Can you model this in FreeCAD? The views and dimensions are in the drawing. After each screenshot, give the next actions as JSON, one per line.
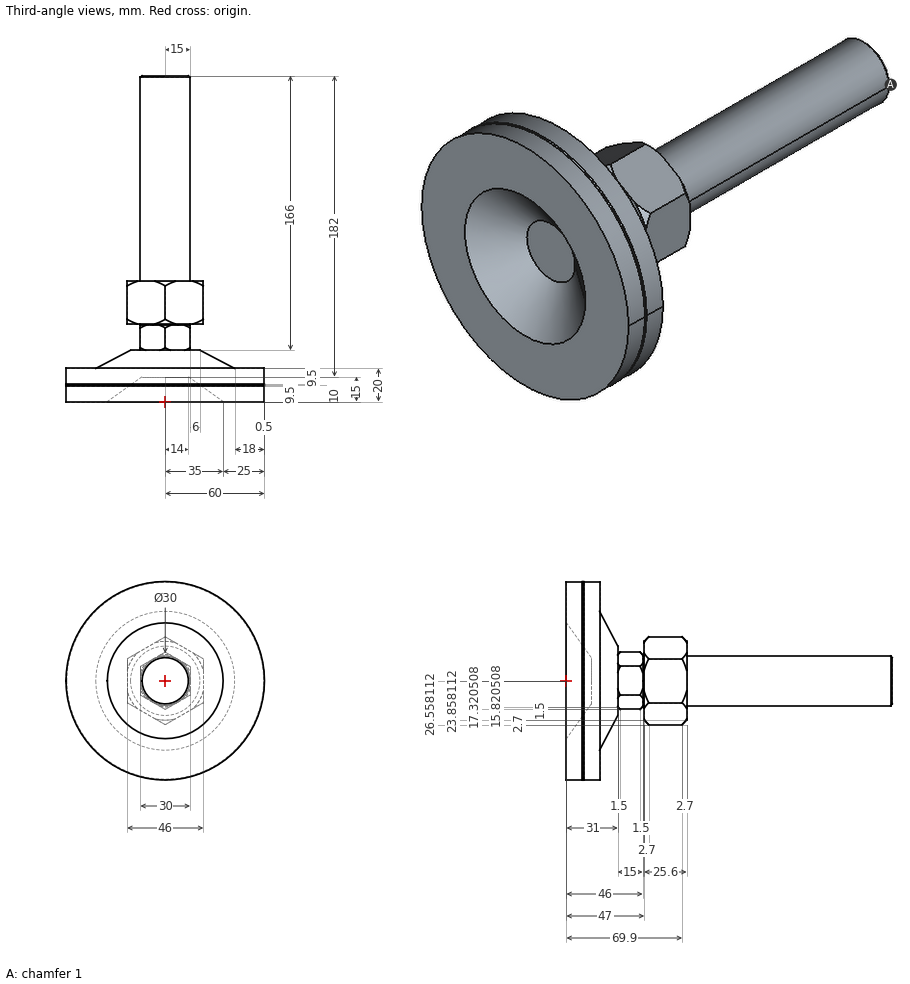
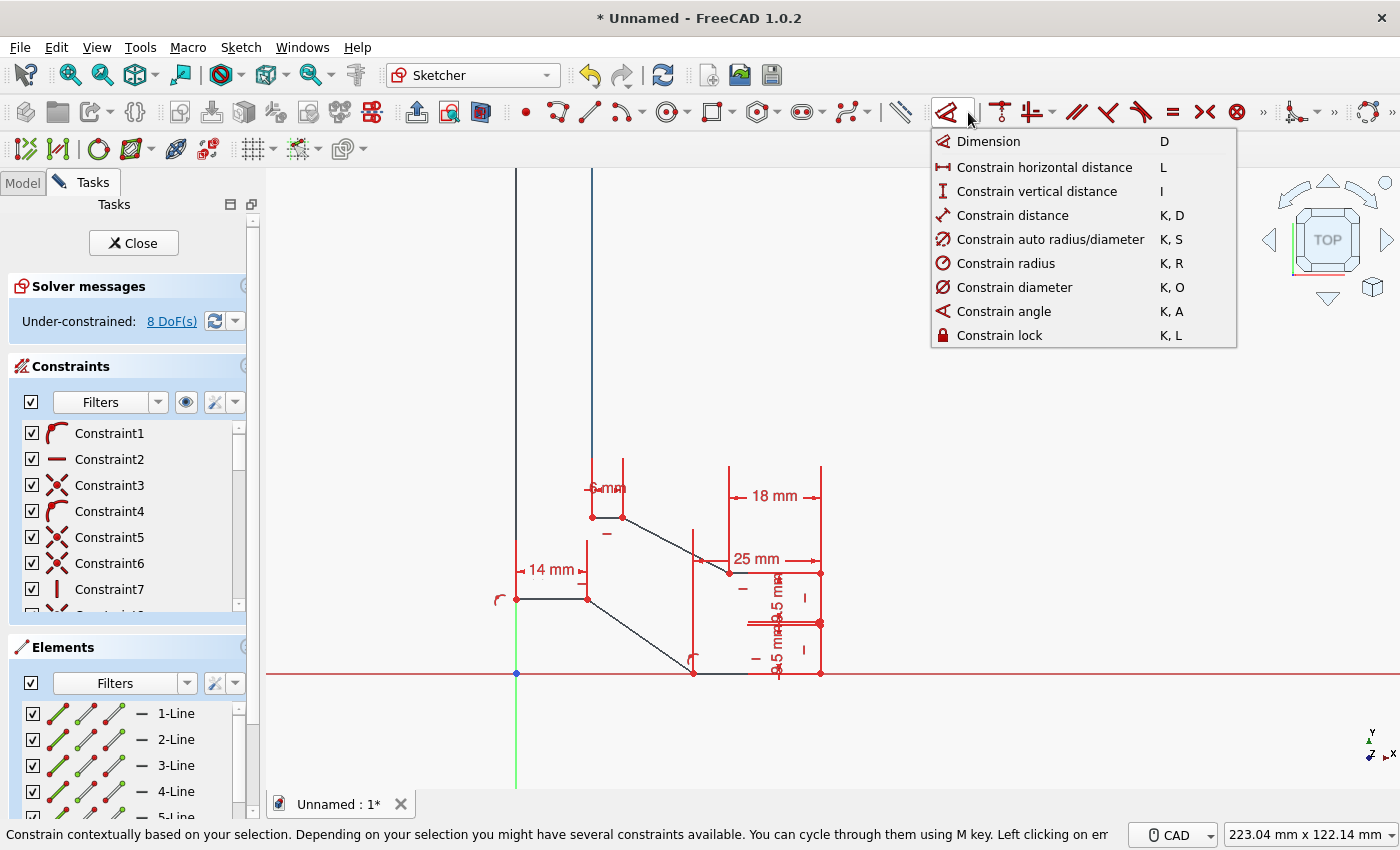
{"action": "left_click", "coordinate": [1084, 191]}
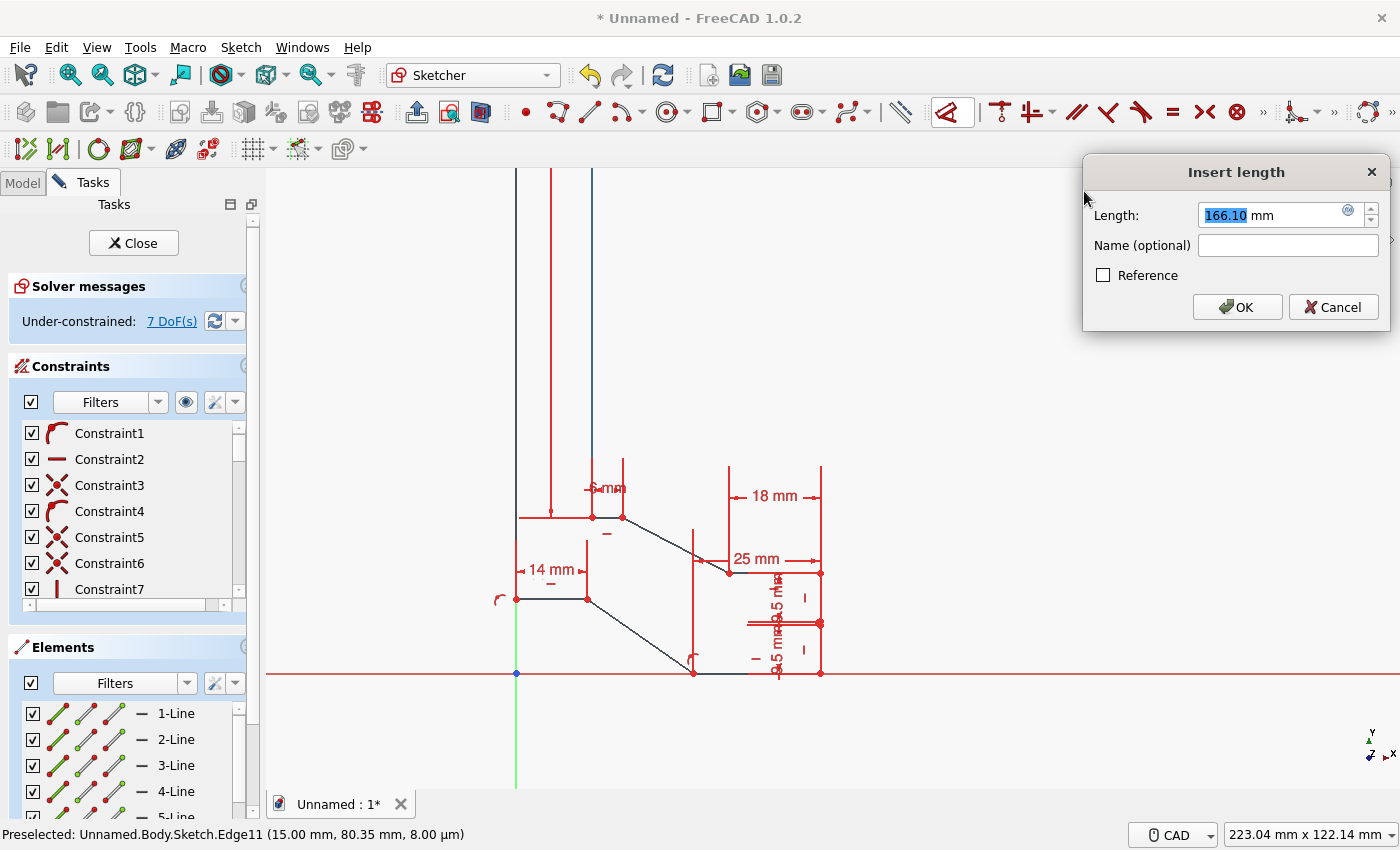
{"action": "type", "text": "166"}
{"action": "key", "text": "Return"}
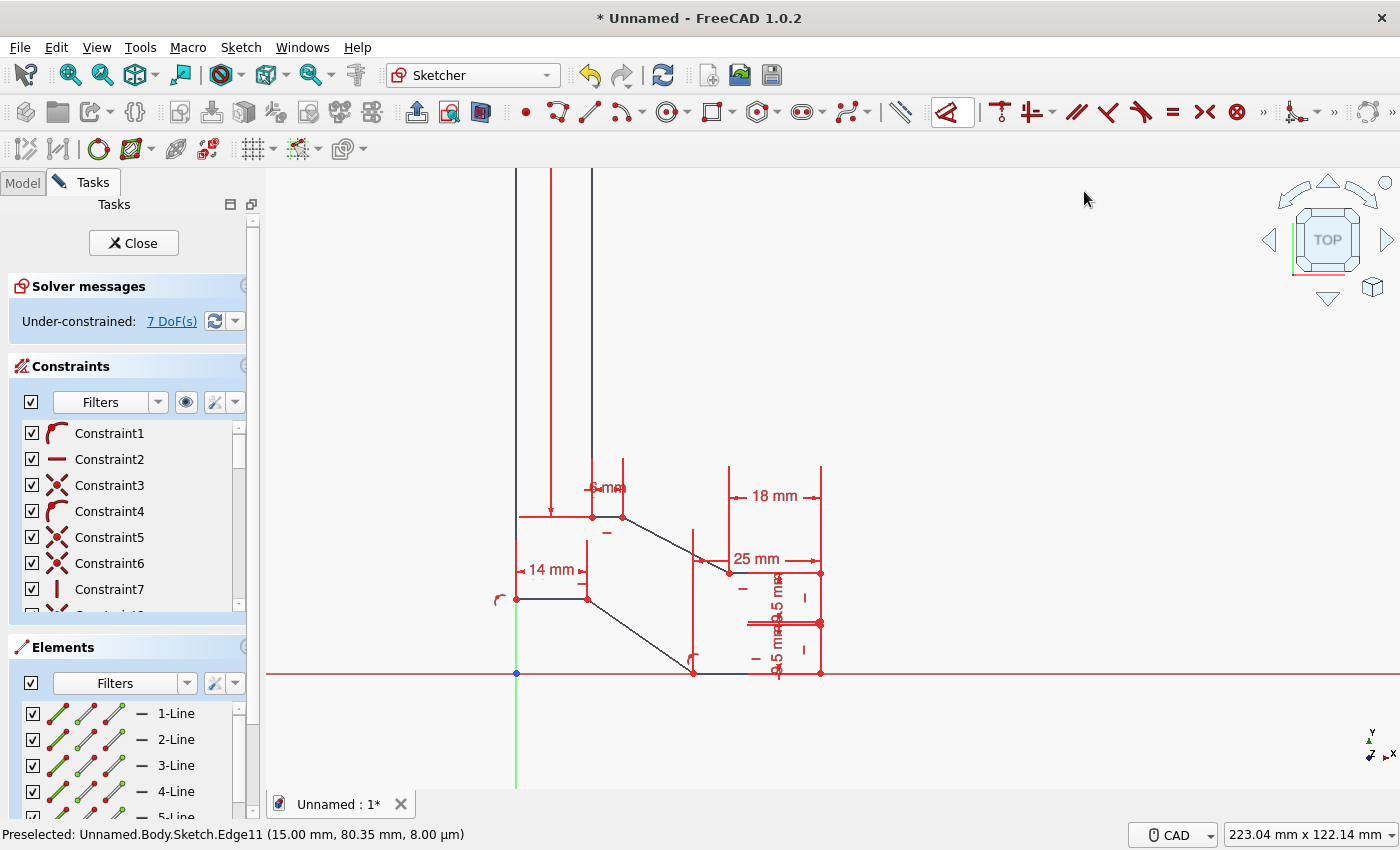
{"action": "left_click", "coordinate": [516, 322]}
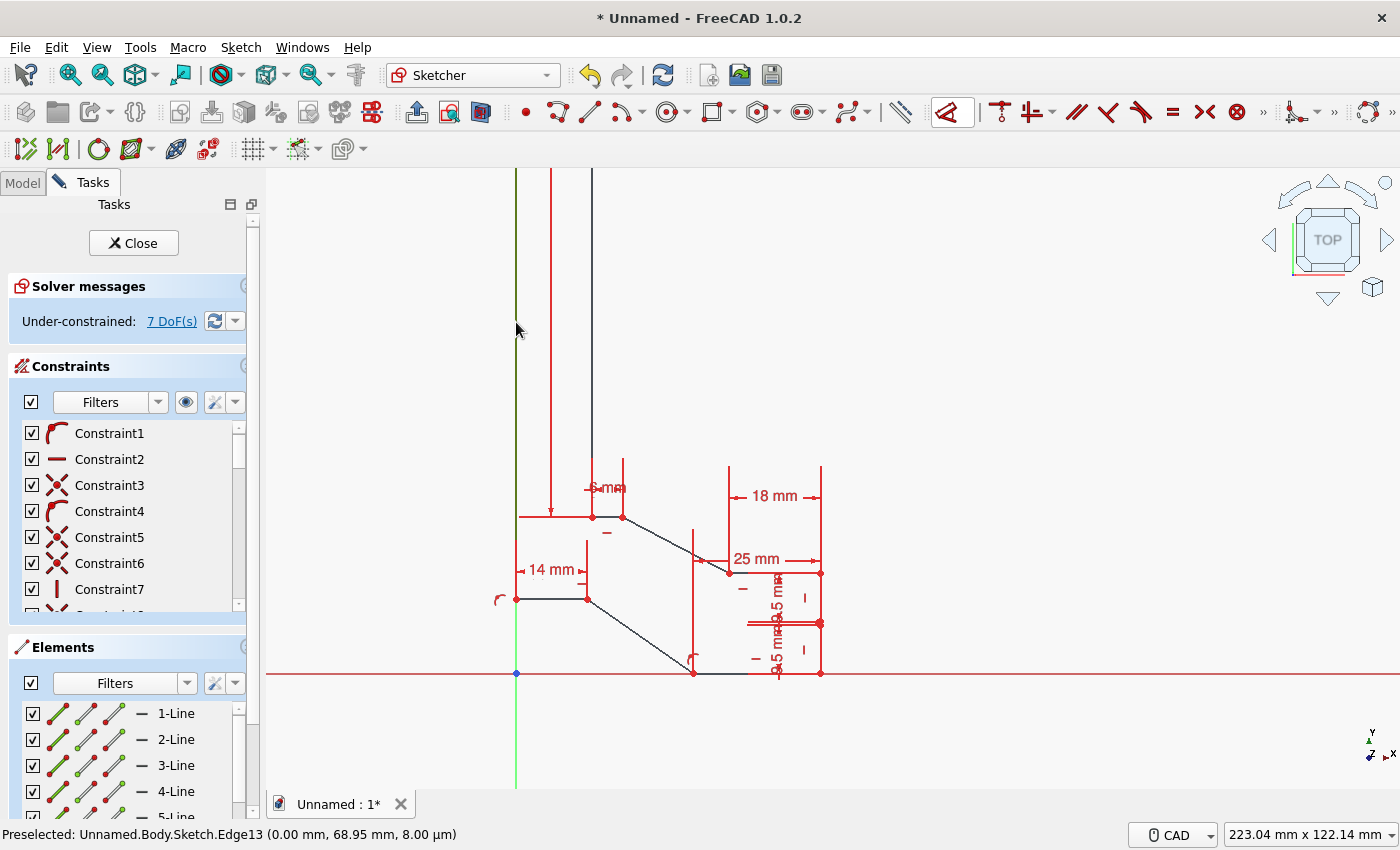
{"action": "key", "text": "i"}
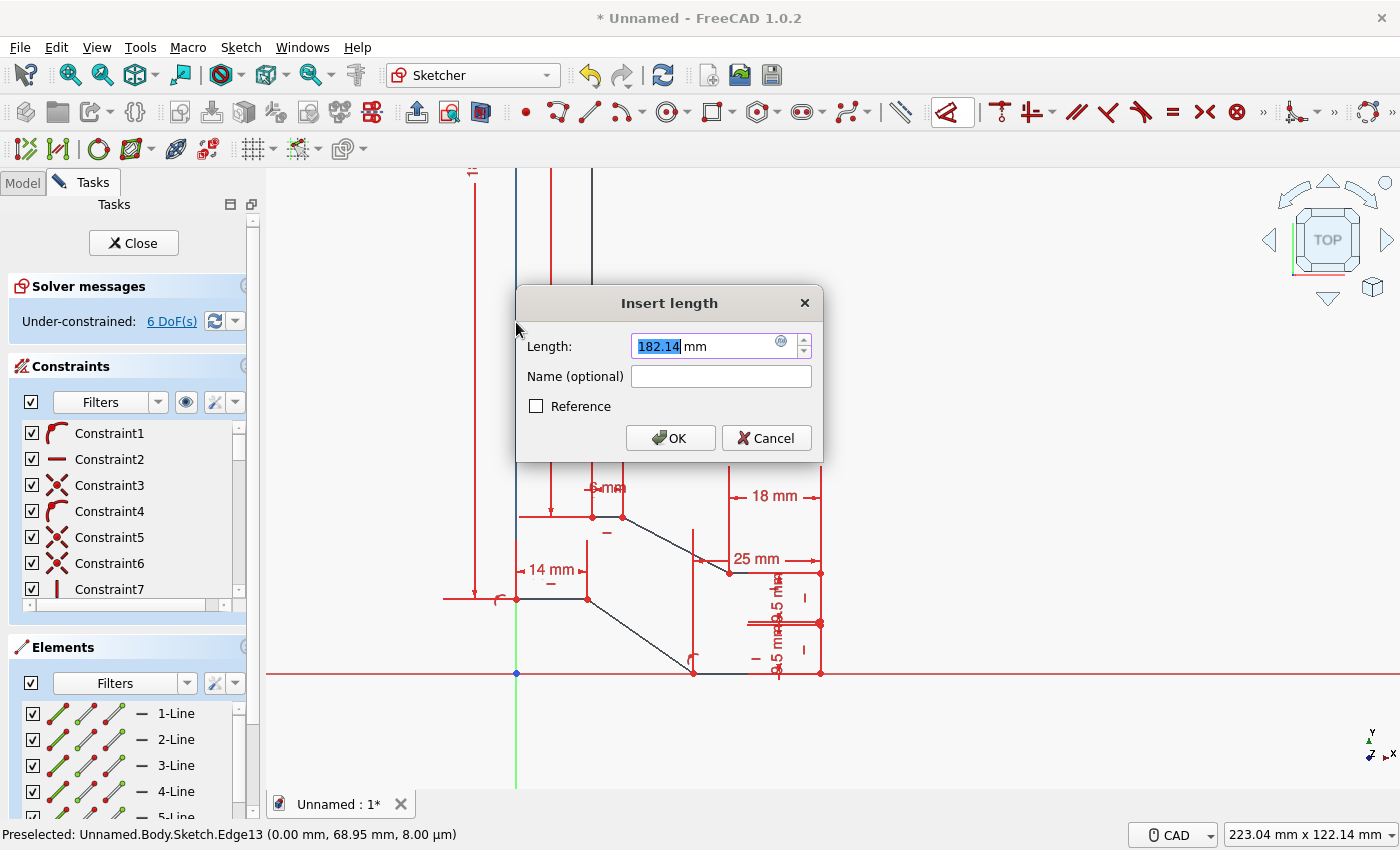
{"action": "type", "text": "182"}
{"action": "key", "text": "Return"}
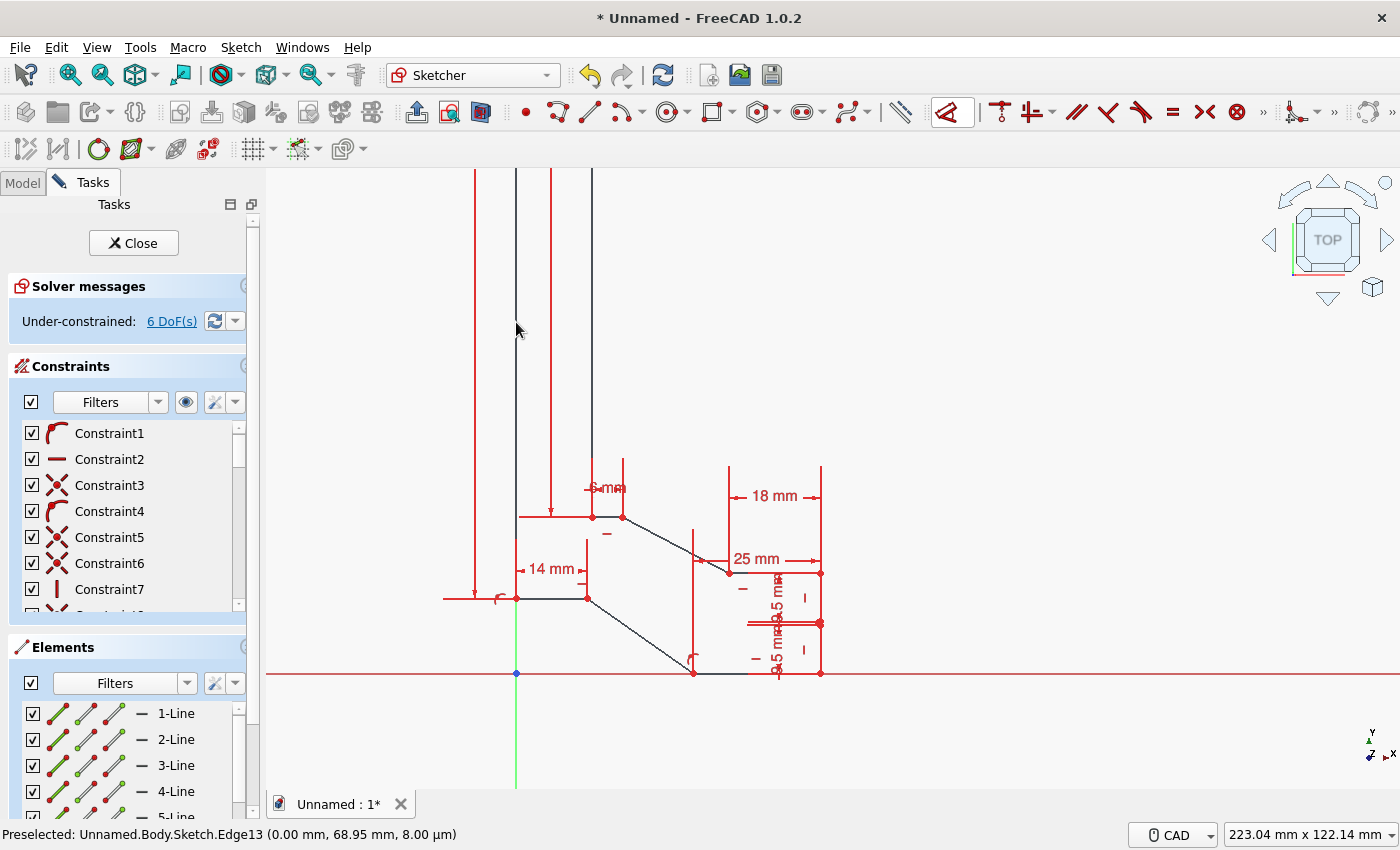
{"action": "left_click", "coordinate": [516, 599]}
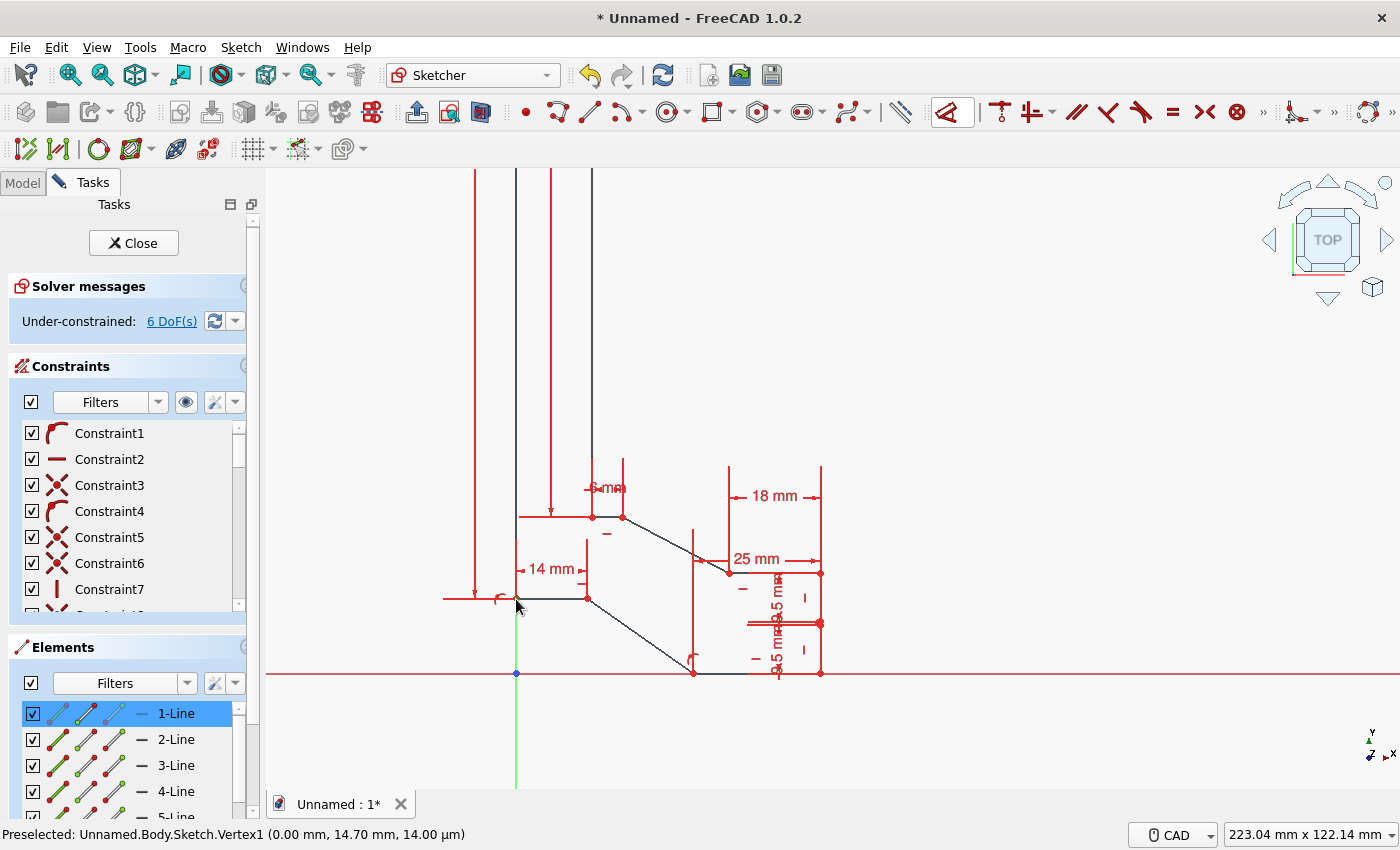
{"action": "key", "text": "i"}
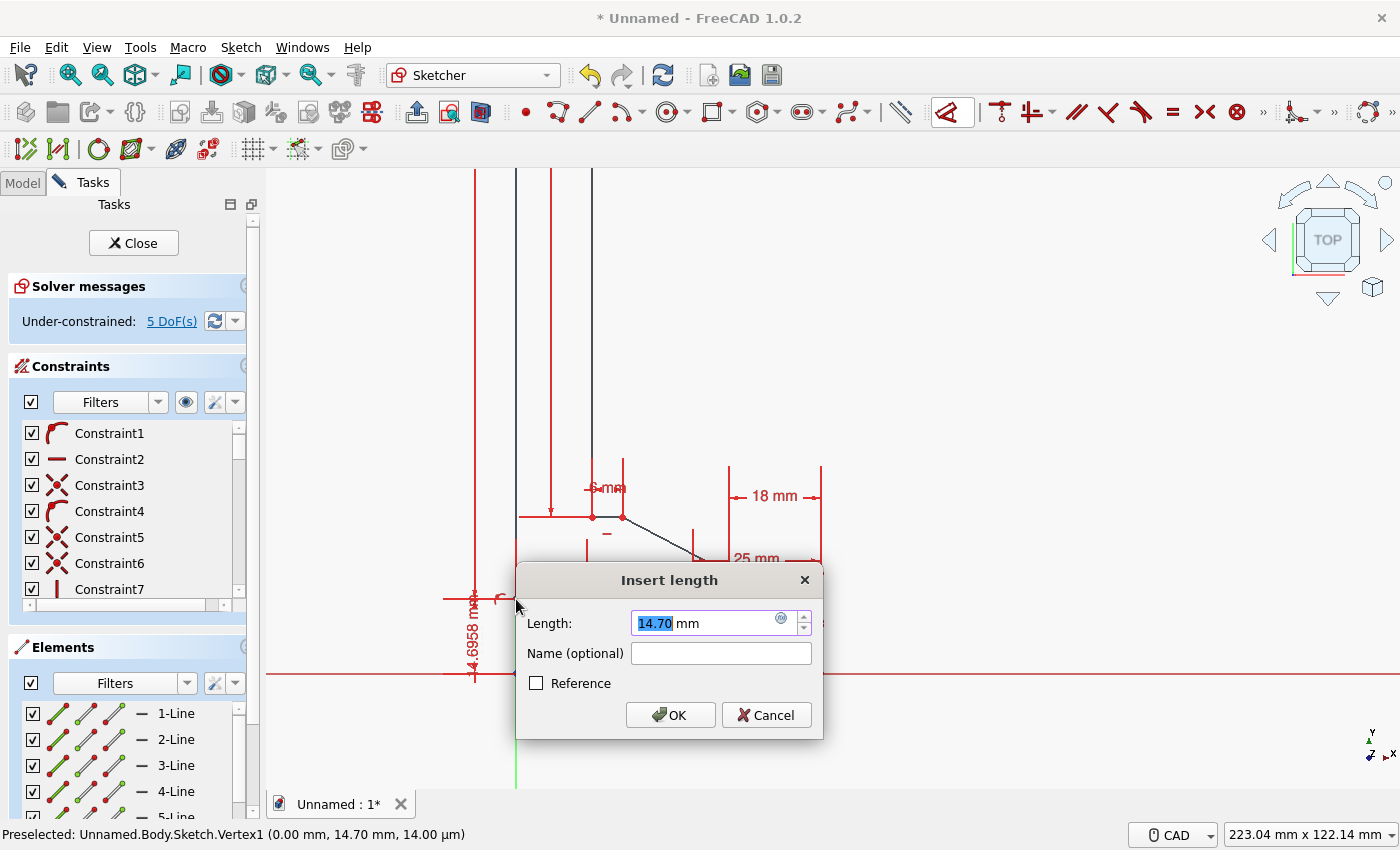
{"action": "type", "text": "15"}
{"action": "key", "text": "Return"}